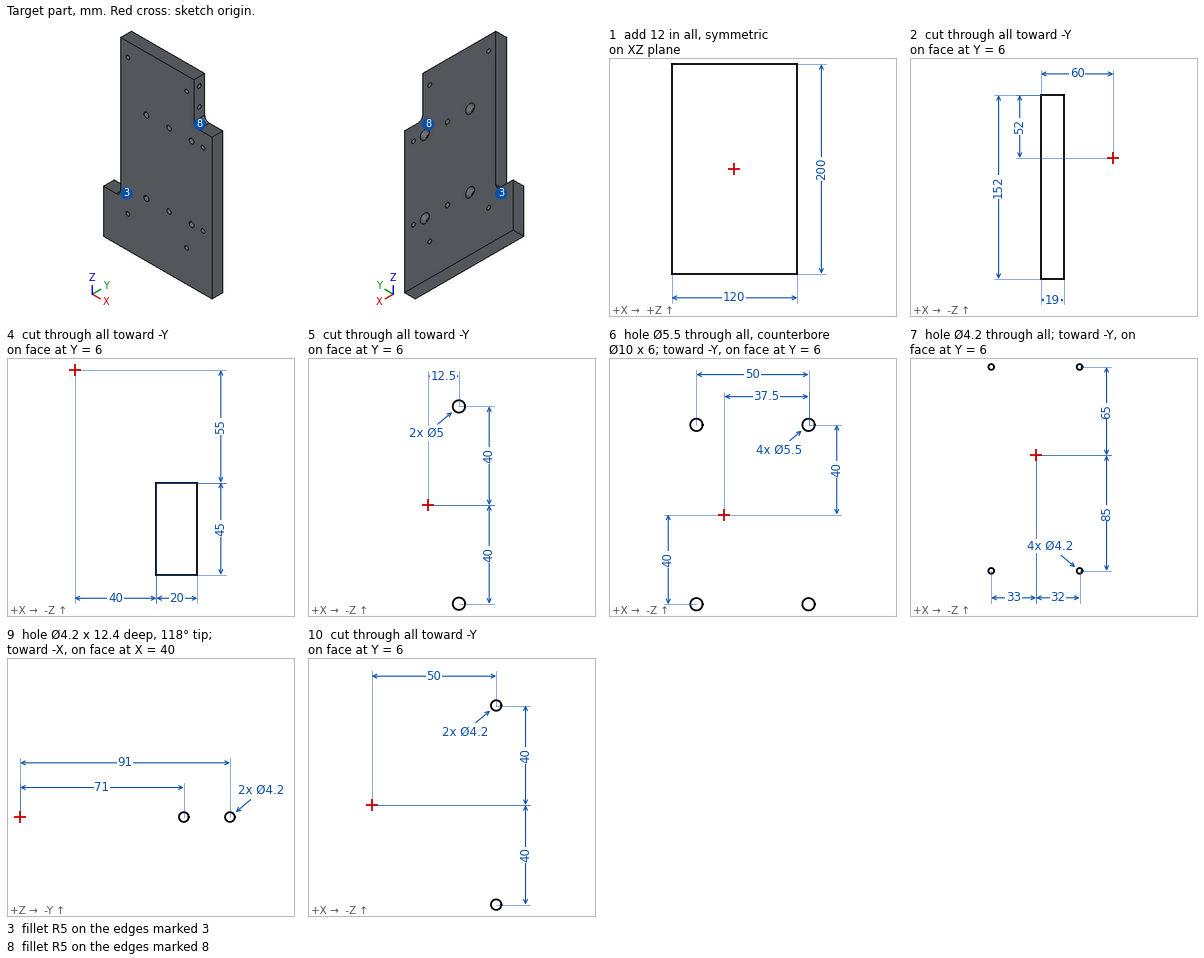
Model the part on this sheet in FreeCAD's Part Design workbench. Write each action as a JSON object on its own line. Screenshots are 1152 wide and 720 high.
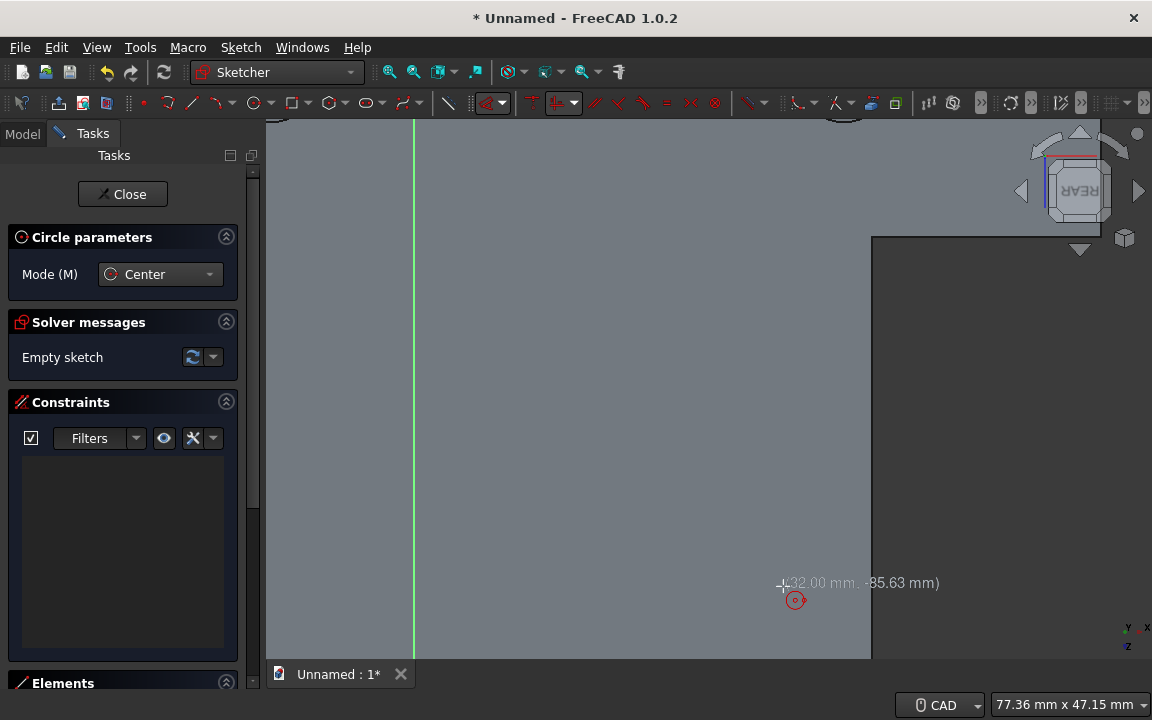
{"action": "scroll", "coordinate": [699, 558], "scroll_direction": "down", "scroll_amount": 8}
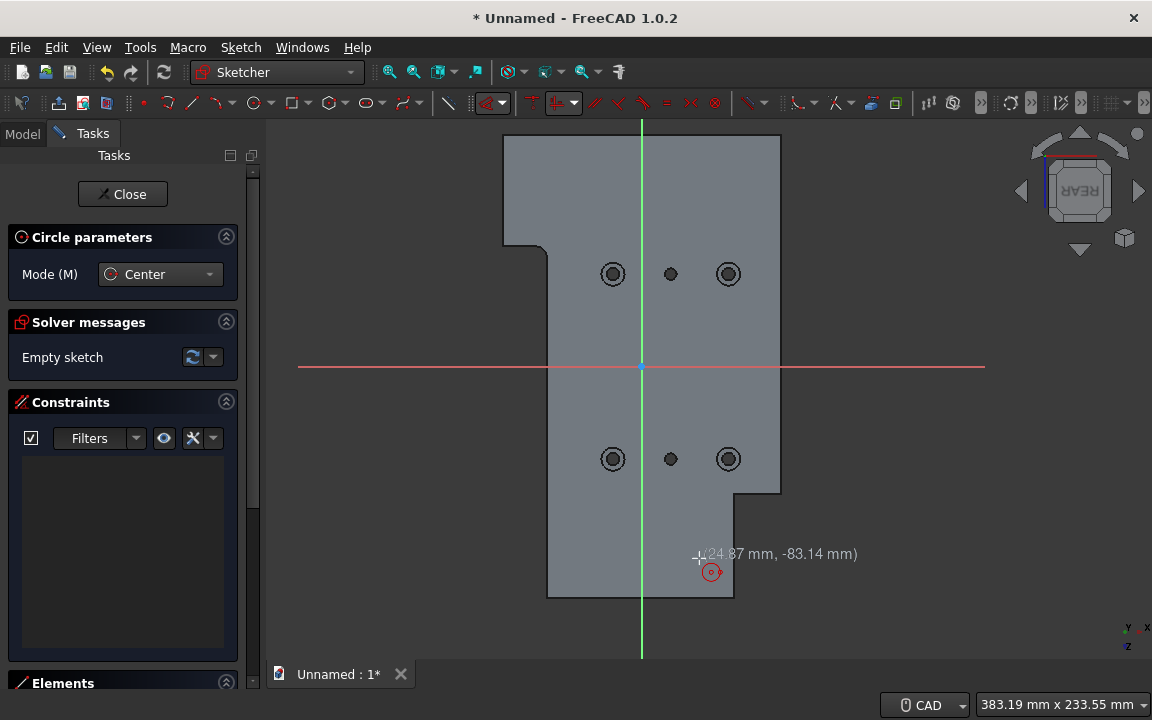
{"action": "left_click", "coordinate": [716, 563]}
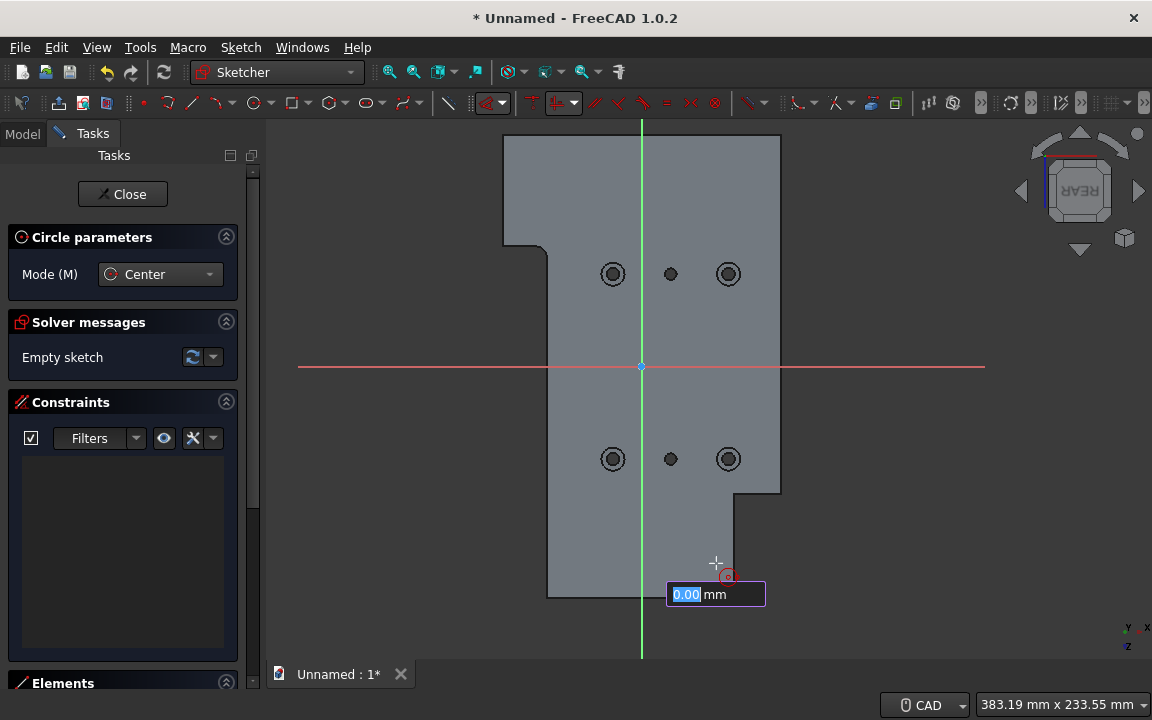
{"action": "scroll", "coordinate": [719, 560], "scroll_direction": "up", "scroll_amount": 6}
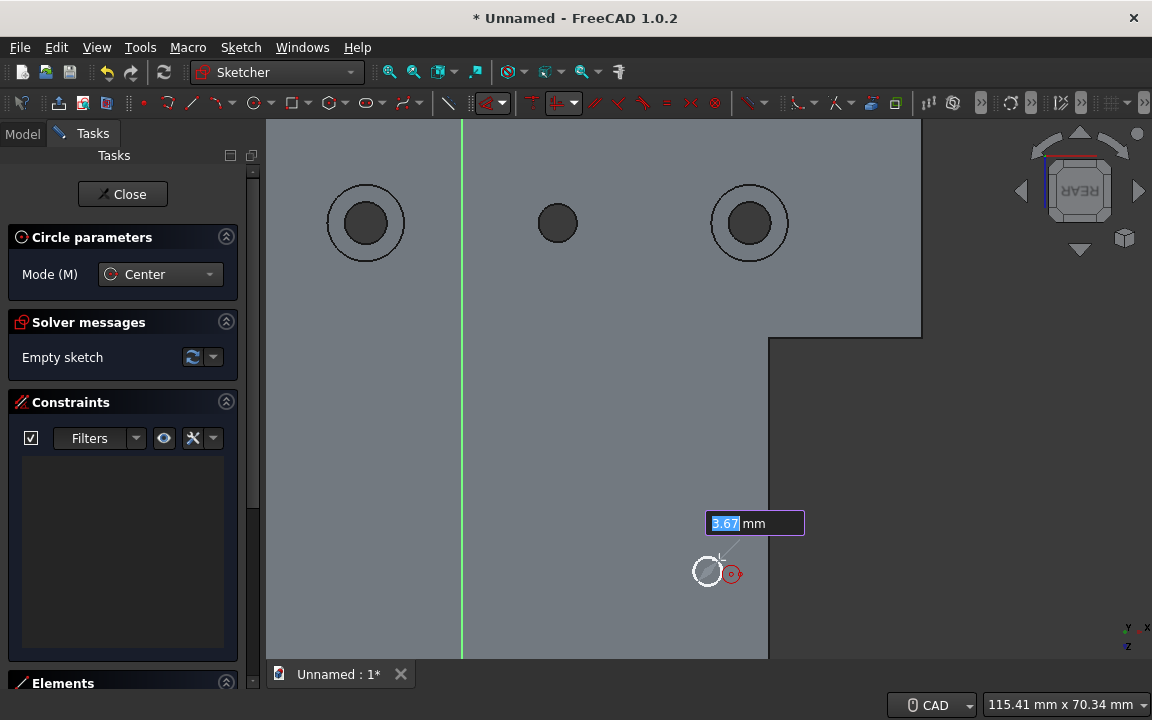
{"action": "left_click", "coordinate": [719, 557]}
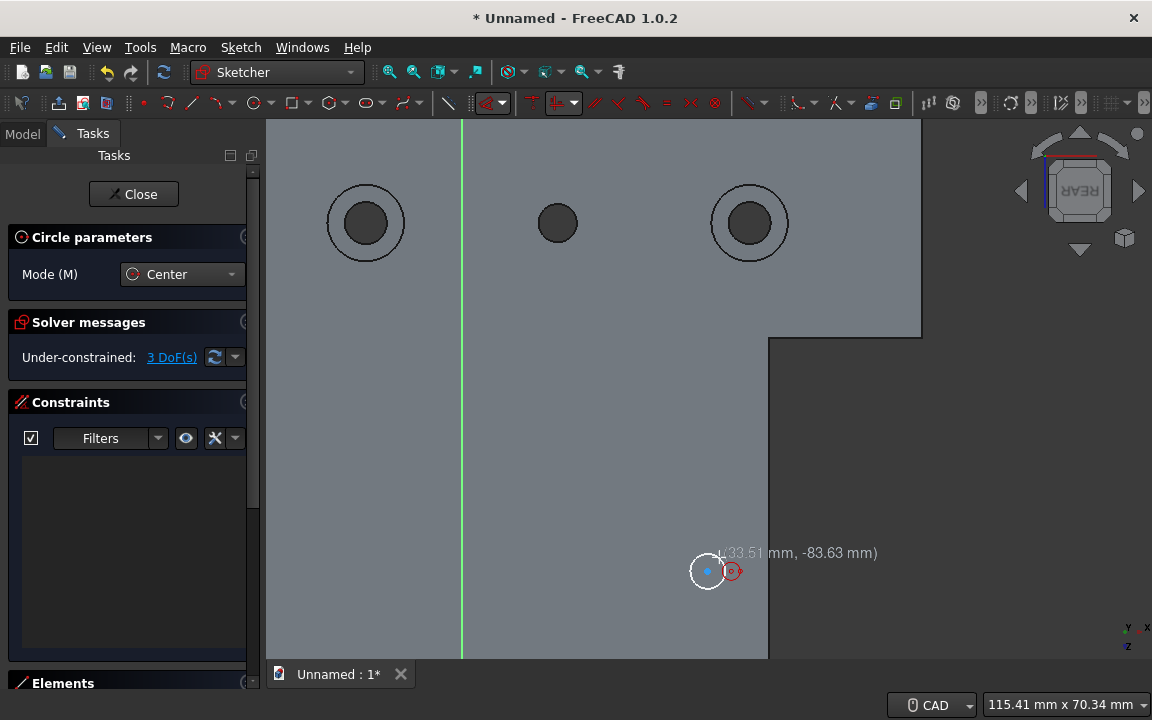
{"action": "scroll", "coordinate": [719, 560], "scroll_direction": "down", "scroll_amount": 6}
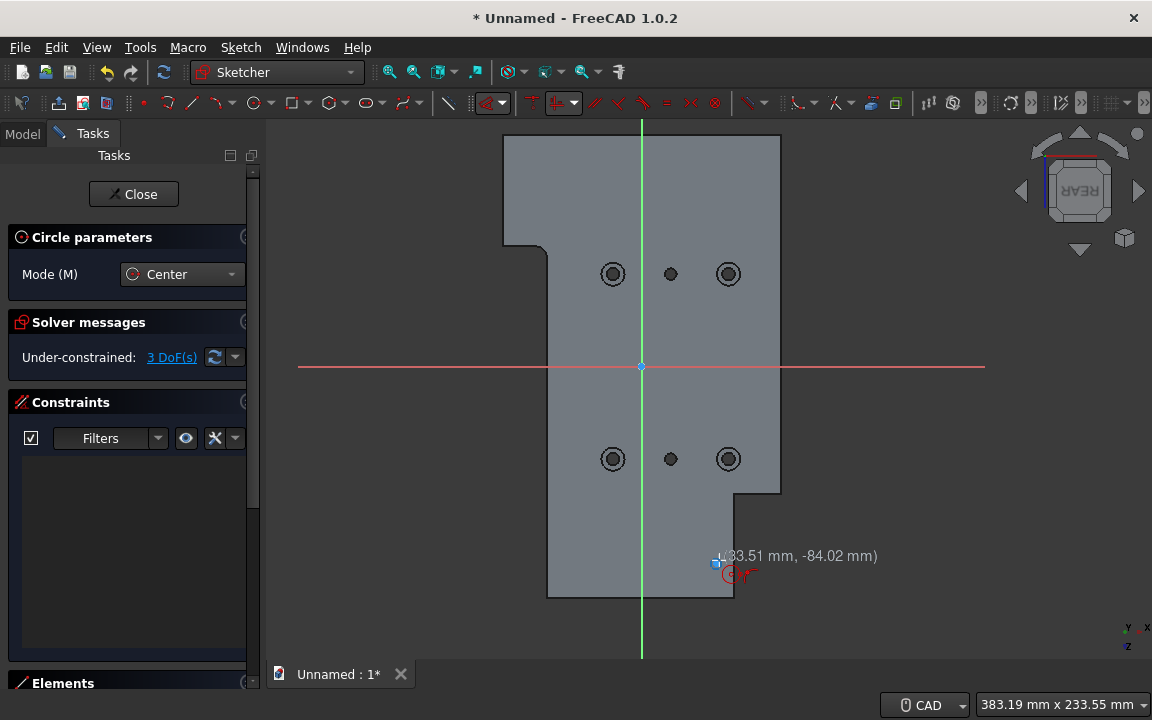
{"action": "scroll", "coordinate": [566, 563], "scroll_direction": "up", "scroll_amount": 8}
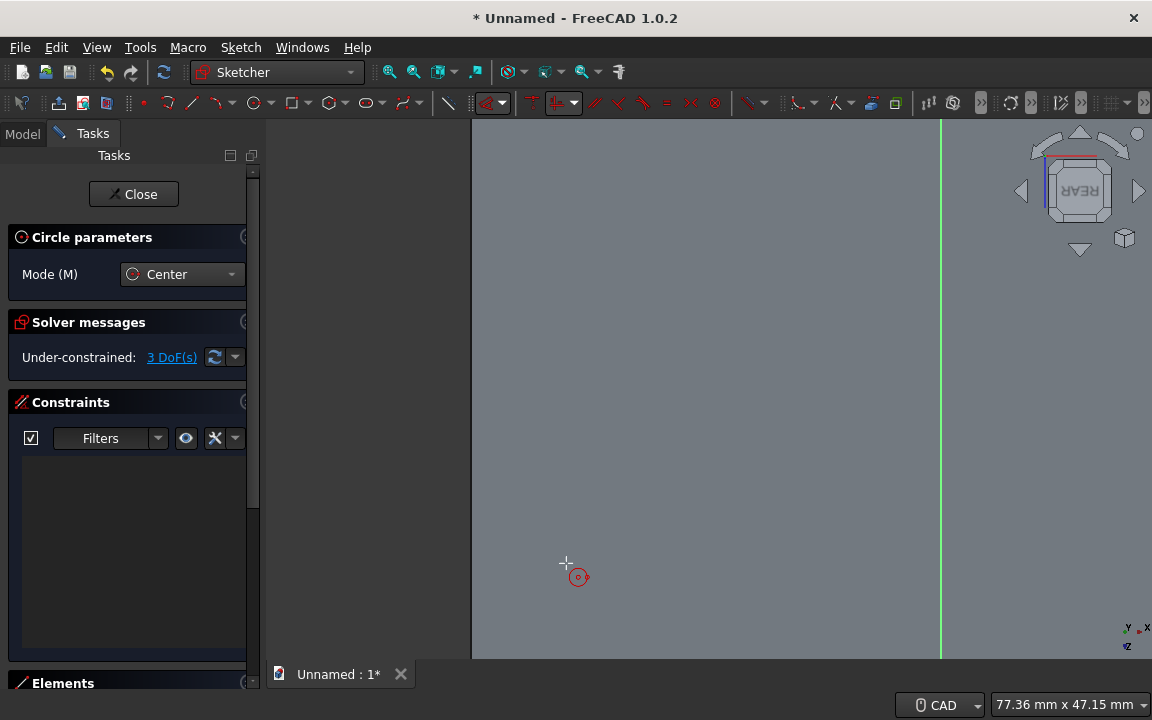
{"action": "scroll", "coordinate": [566, 563], "scroll_direction": "down", "scroll_amount": 8}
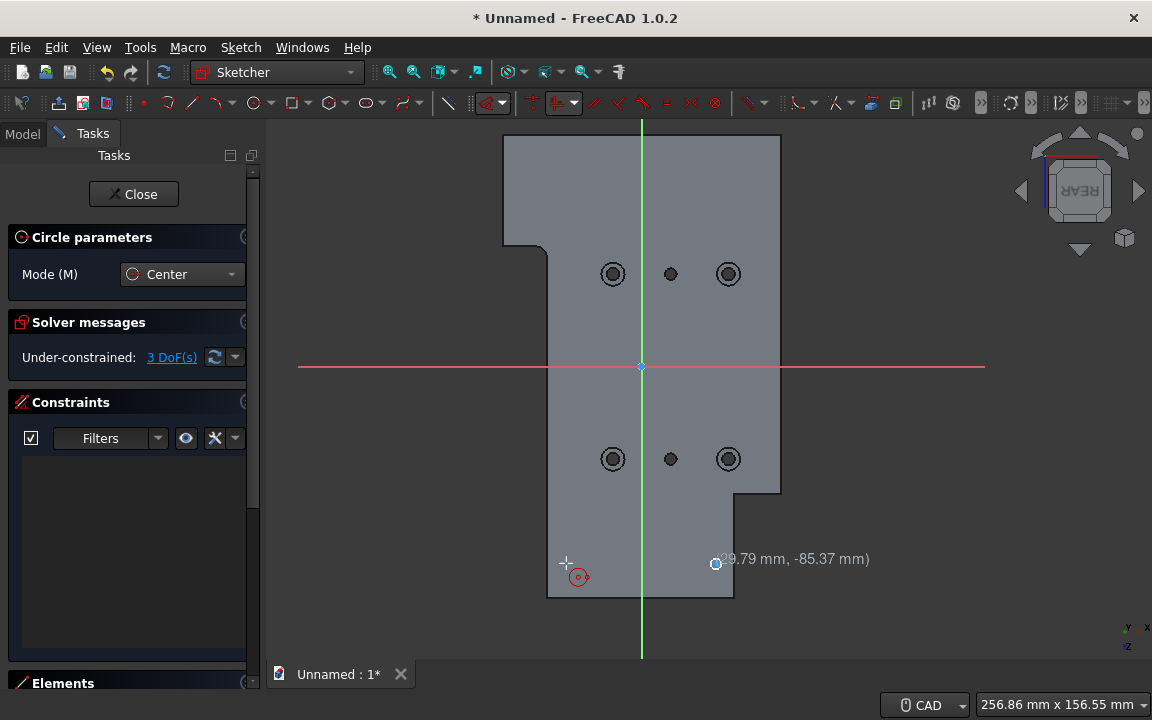
{"action": "left_click", "coordinate": [566, 563]}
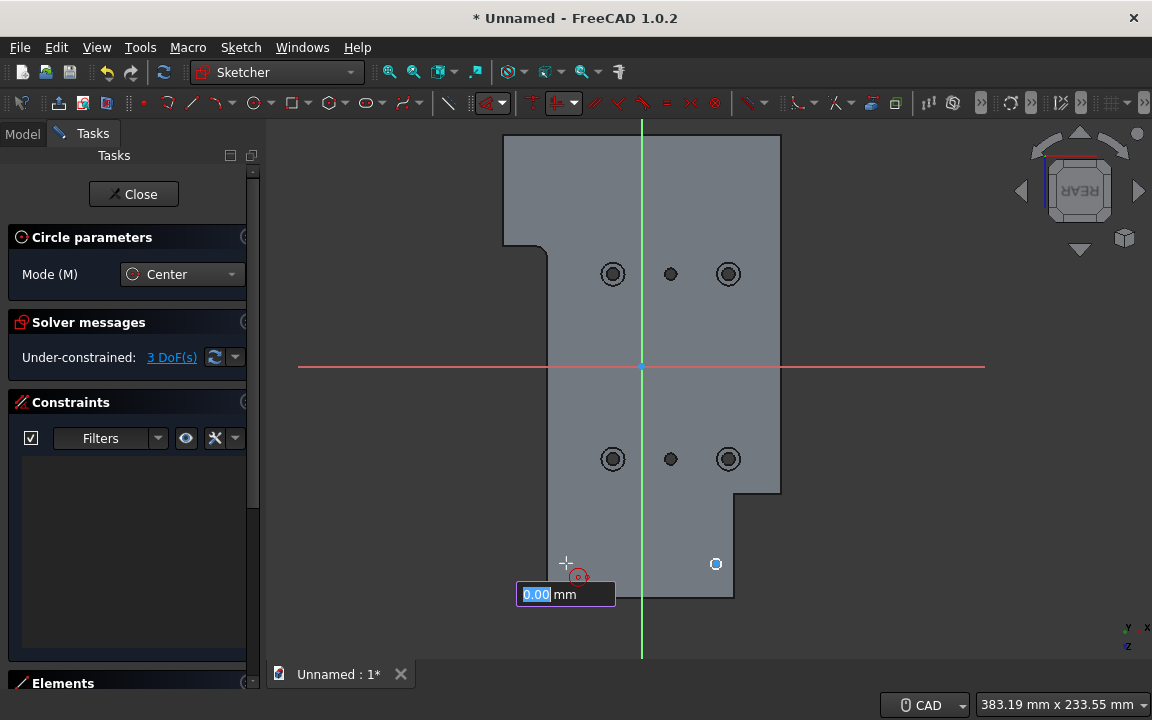
{"action": "scroll", "coordinate": [569, 560], "scroll_direction": "up", "scroll_amount": 6}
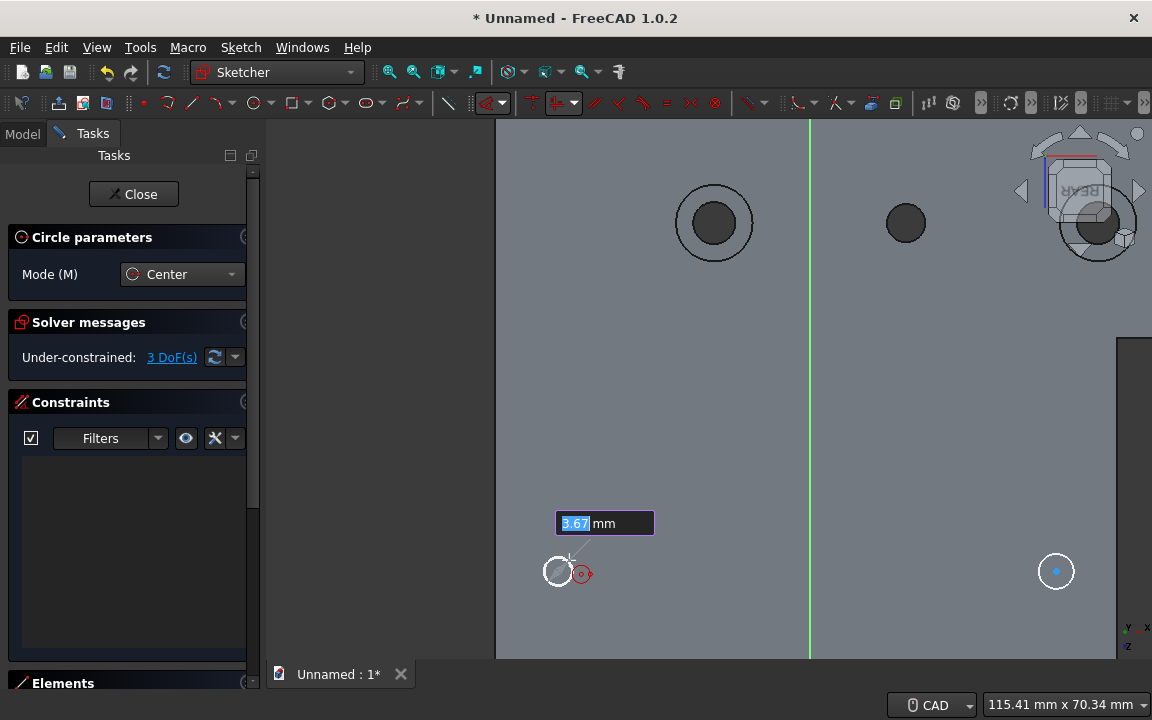
{"action": "left_click", "coordinate": [568, 557]}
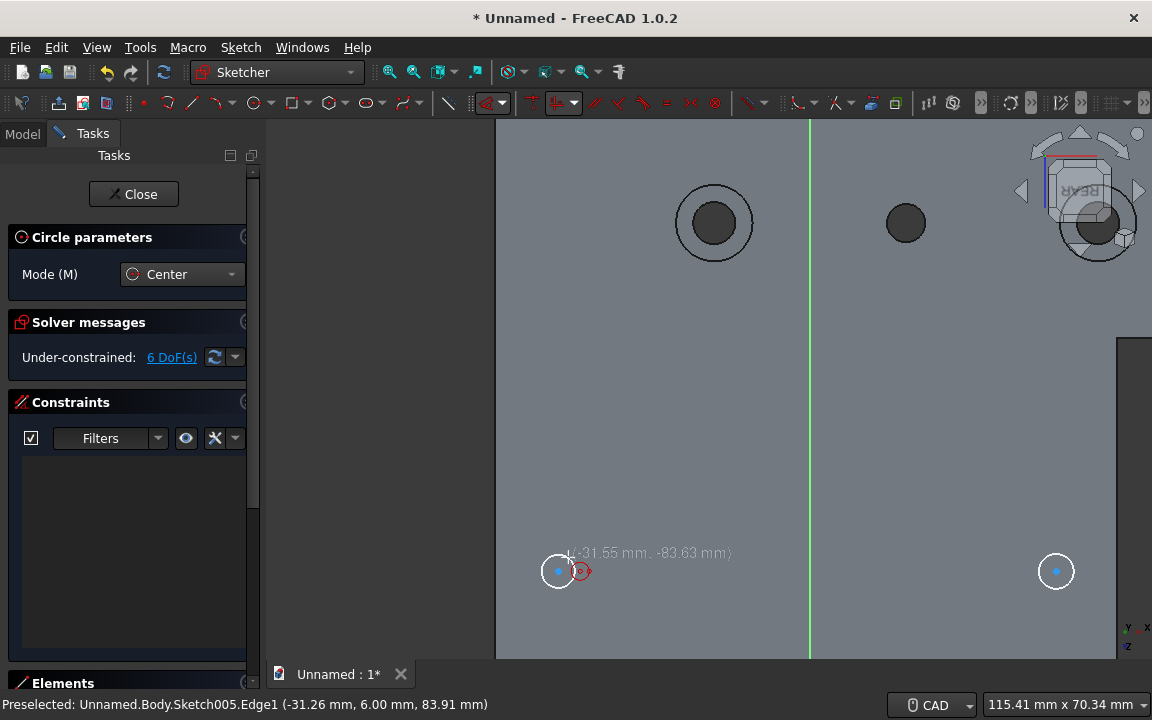
{"action": "scroll", "coordinate": [569, 560], "scroll_direction": "down", "scroll_amount": 6}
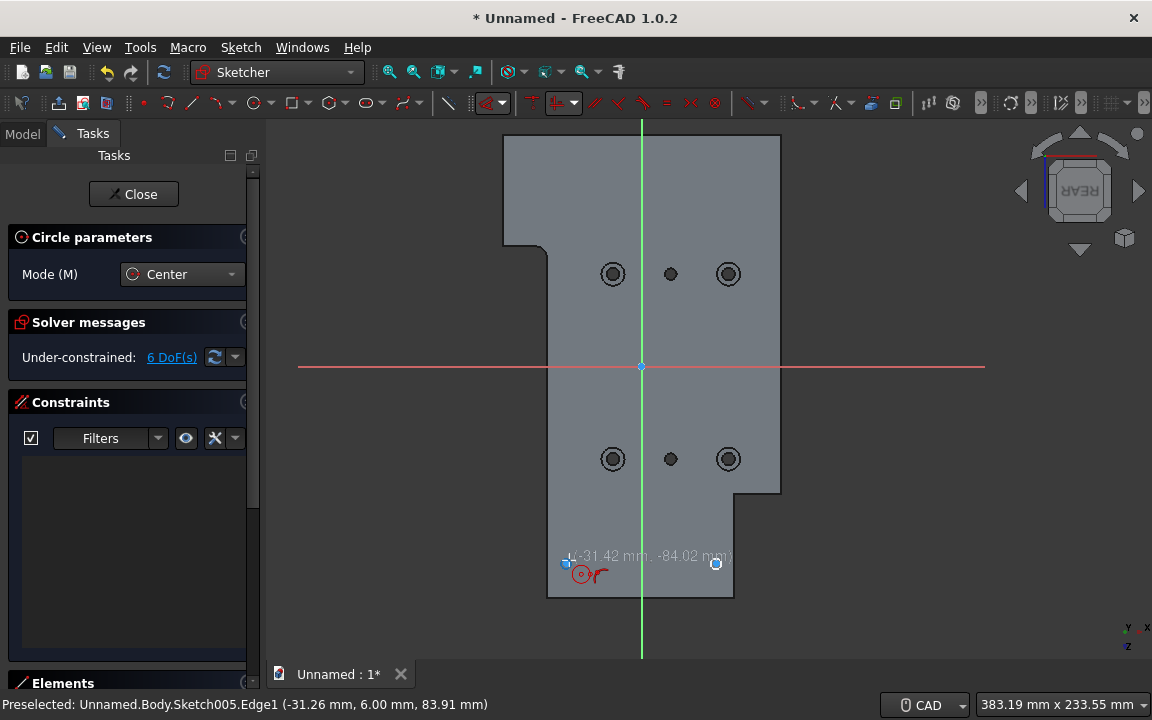
{"action": "scroll", "coordinate": [716, 216], "scroll_direction": "up", "scroll_amount": 8}